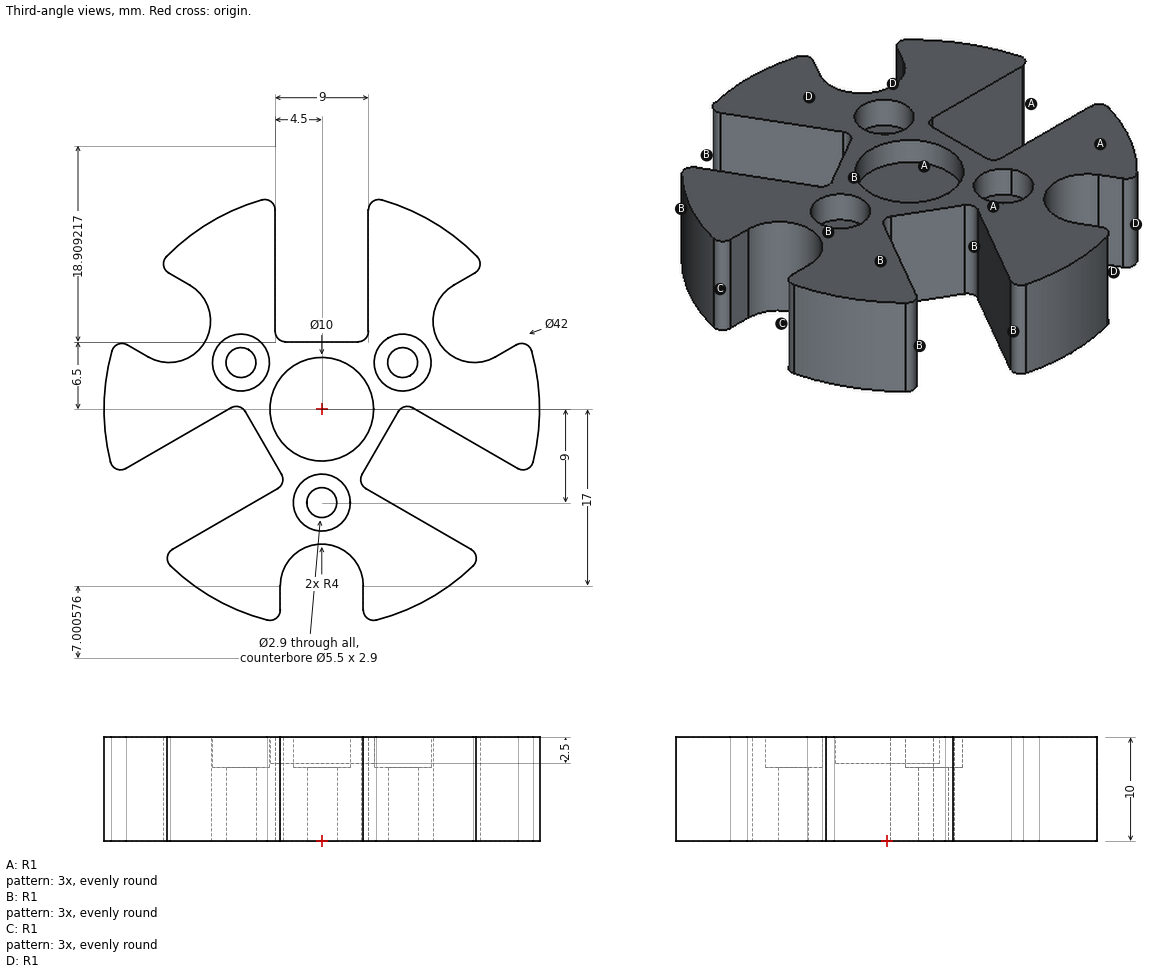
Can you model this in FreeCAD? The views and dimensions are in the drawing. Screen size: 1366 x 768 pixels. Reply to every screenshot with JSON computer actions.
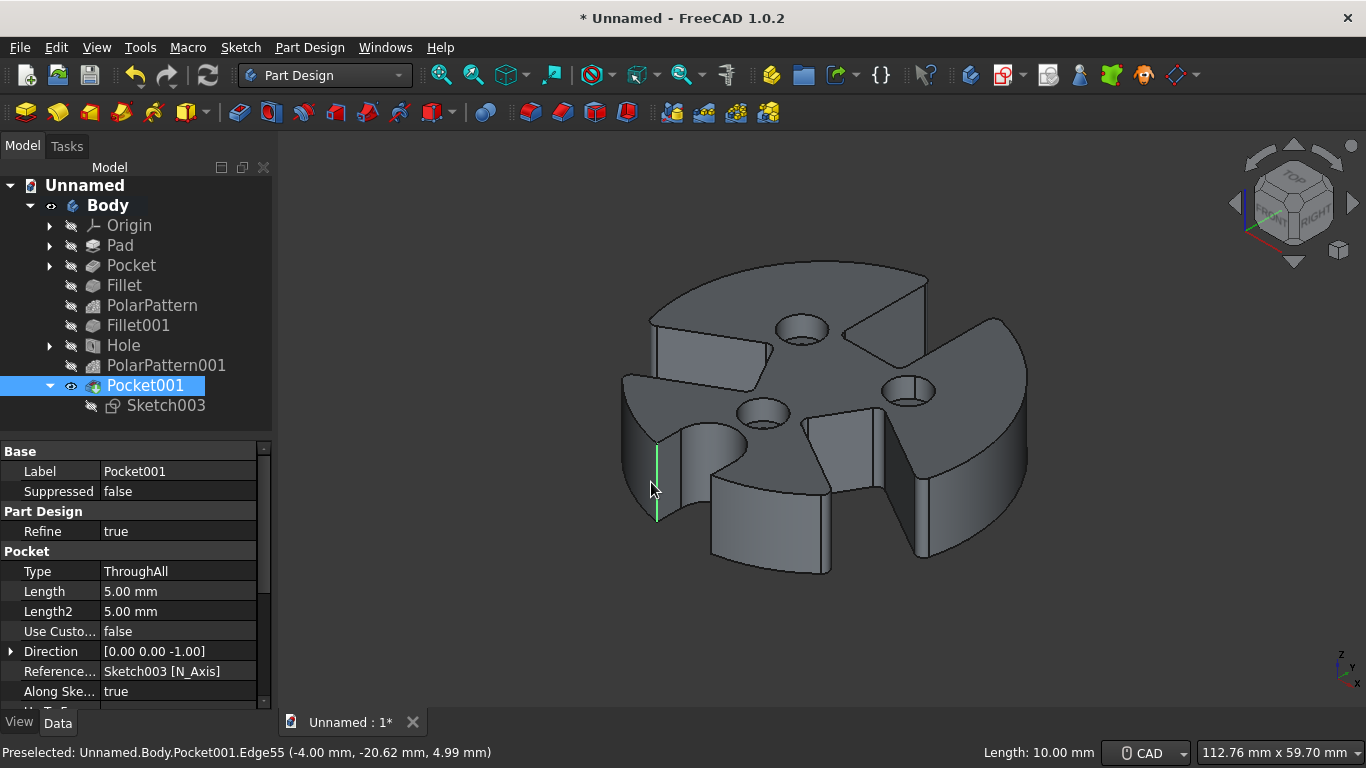
{"action": "key", "text": "2"}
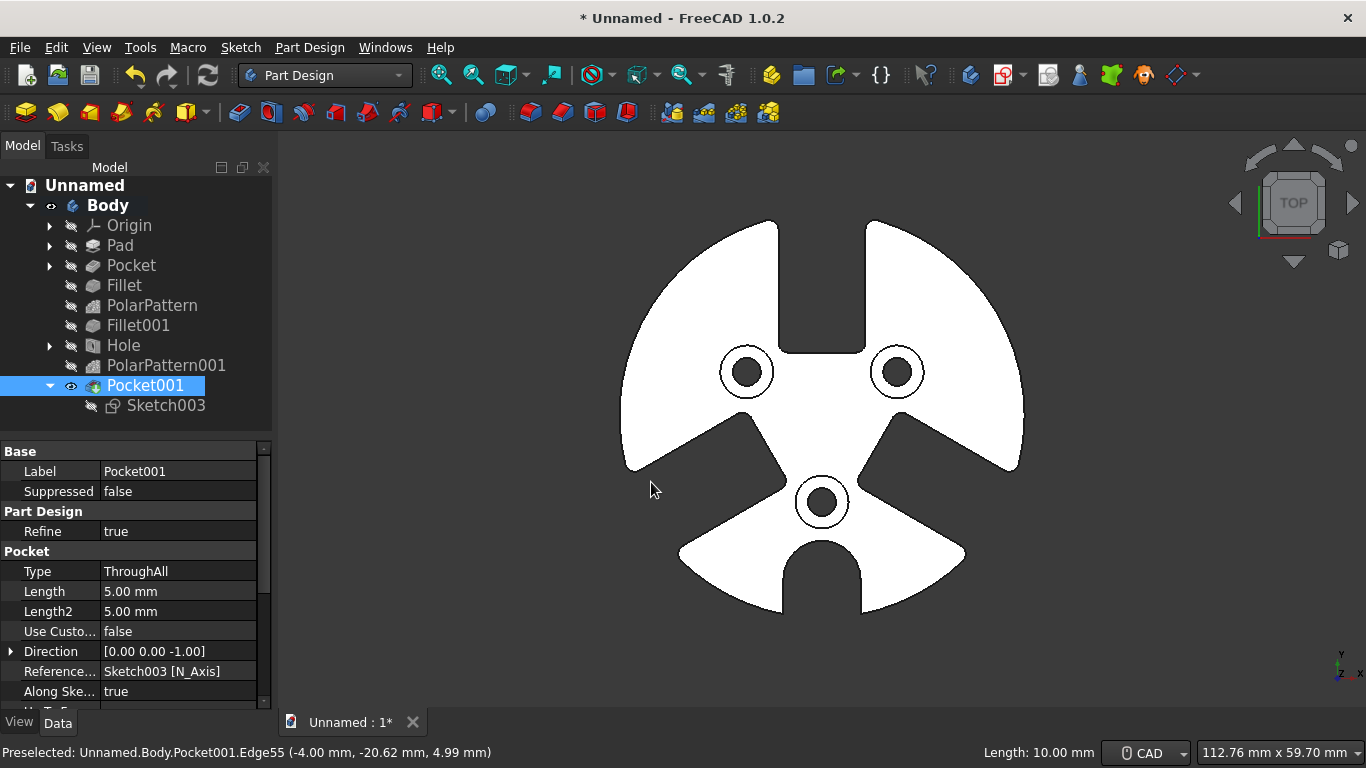
{"action": "key", "text": "0"}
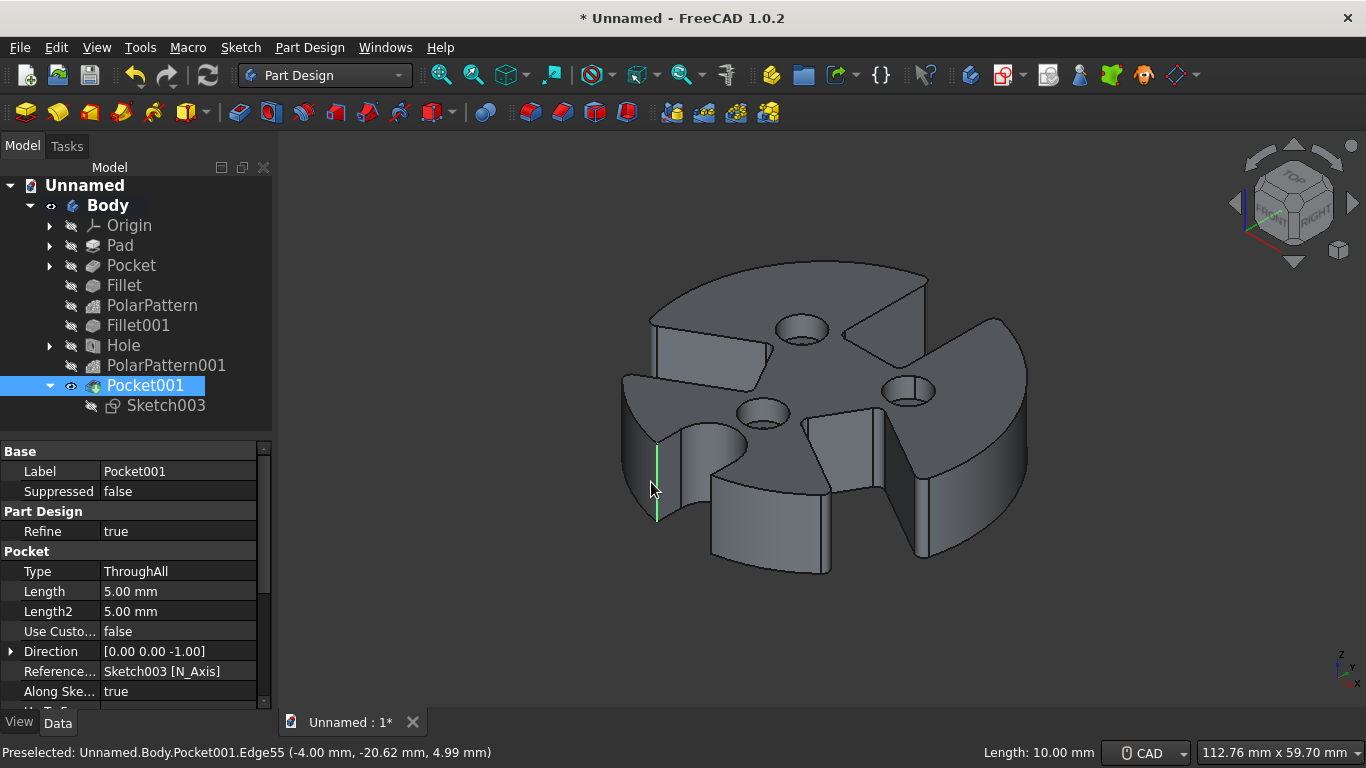
{"action": "key", "text": "1"}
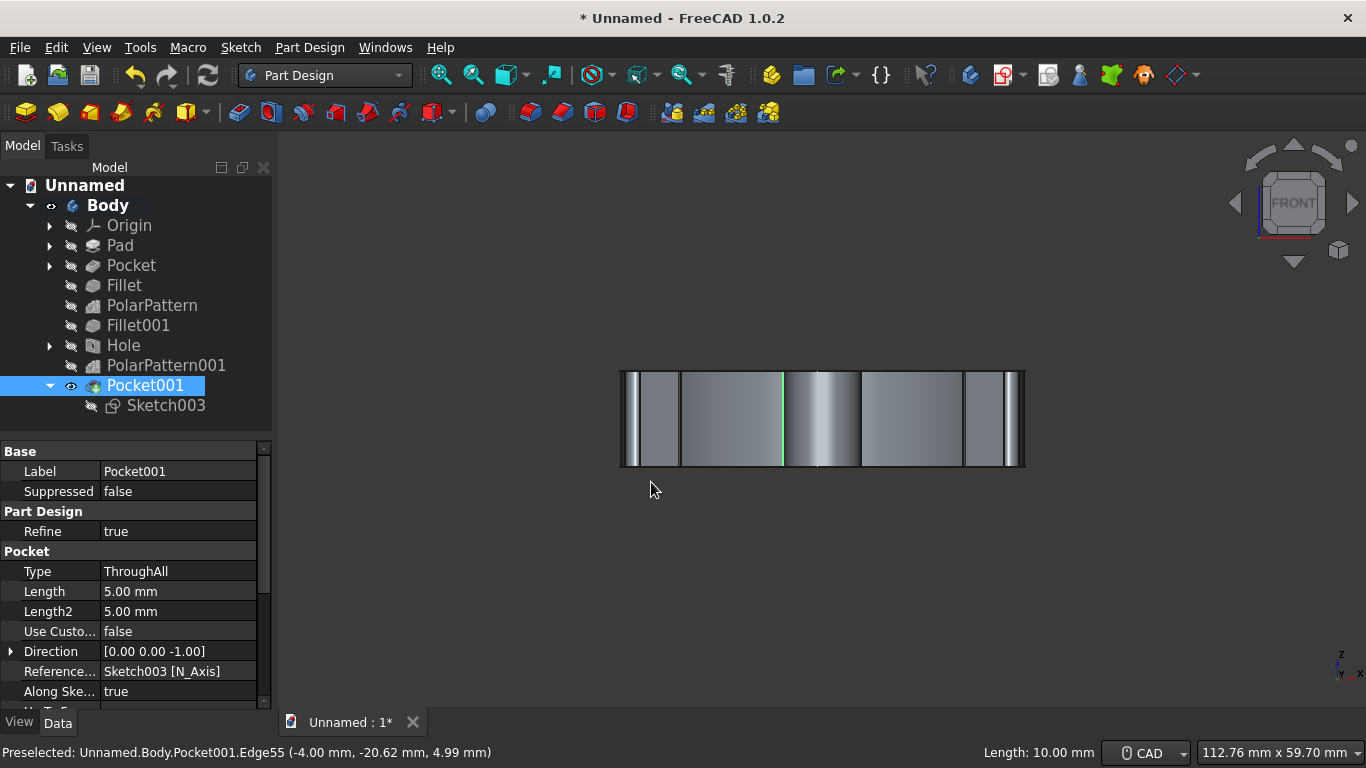
{"action": "left_click", "coordinate": [442, 76]}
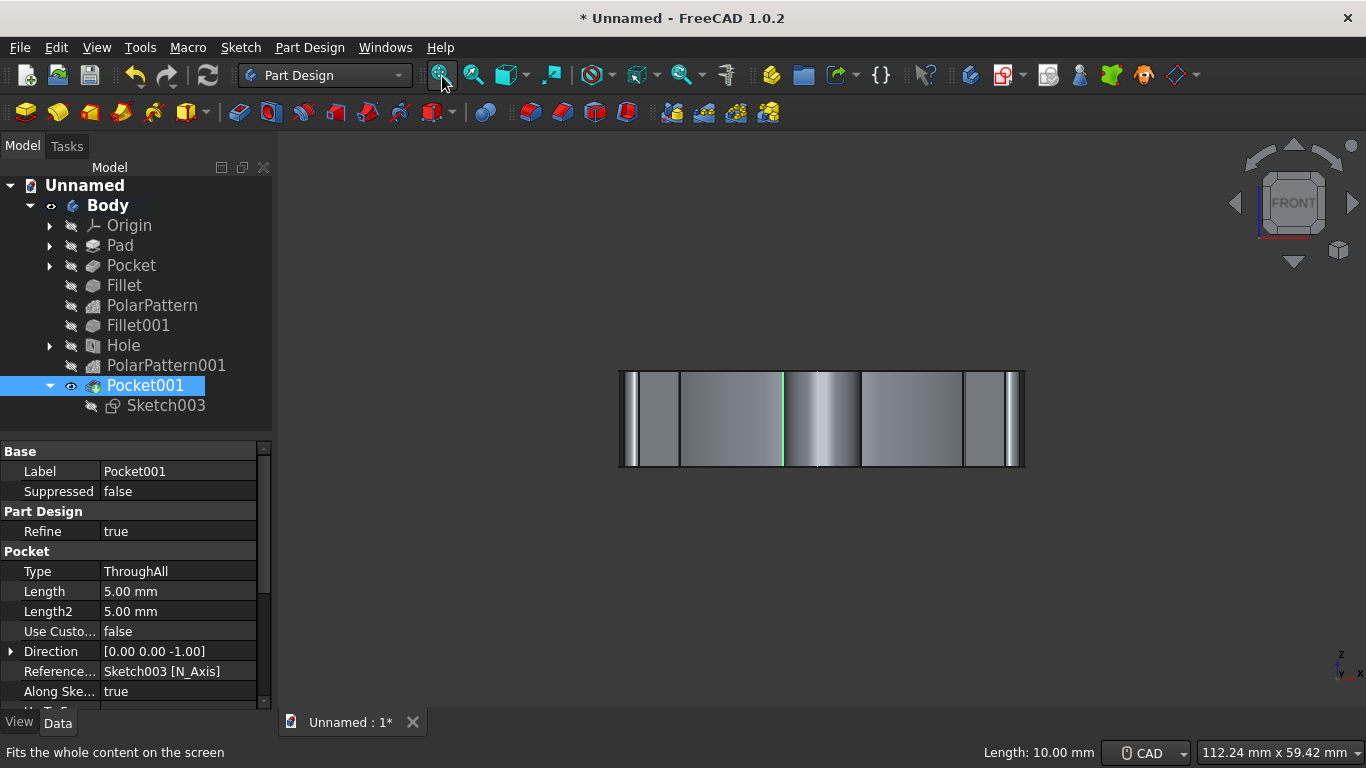
{"action": "left_click", "coordinate": [861, 418], "text": "ctrl"}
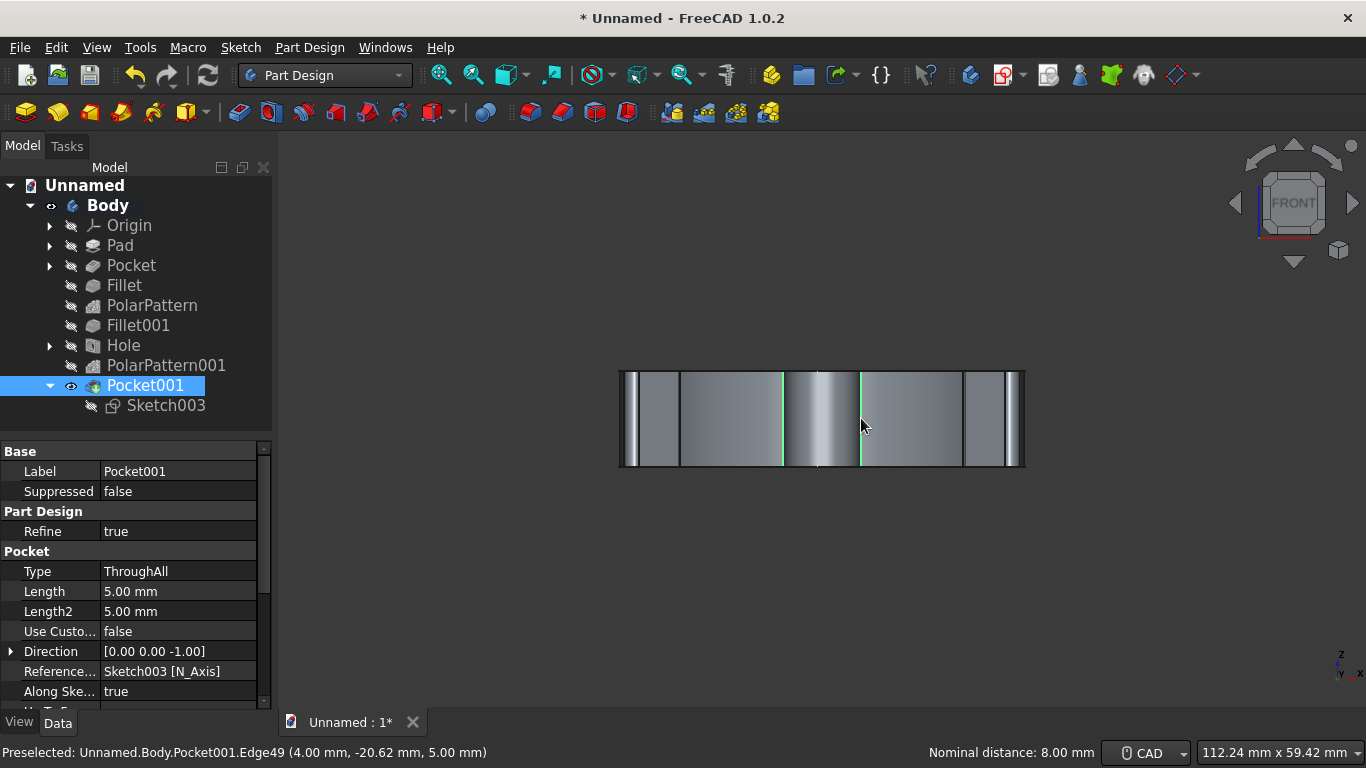
{"action": "left_click", "coordinate": [532, 112]}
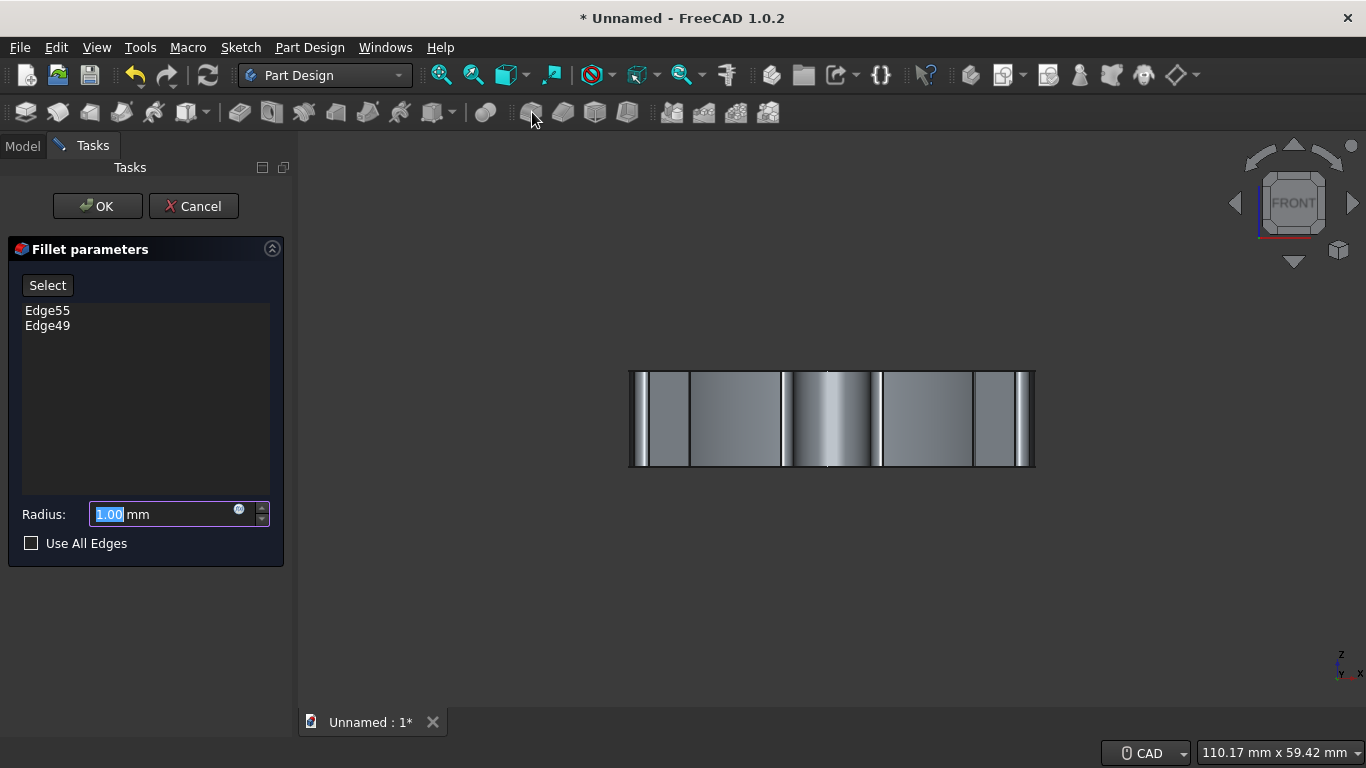
{"action": "type", "text": "1"}
{"action": "key", "text": "Tab"}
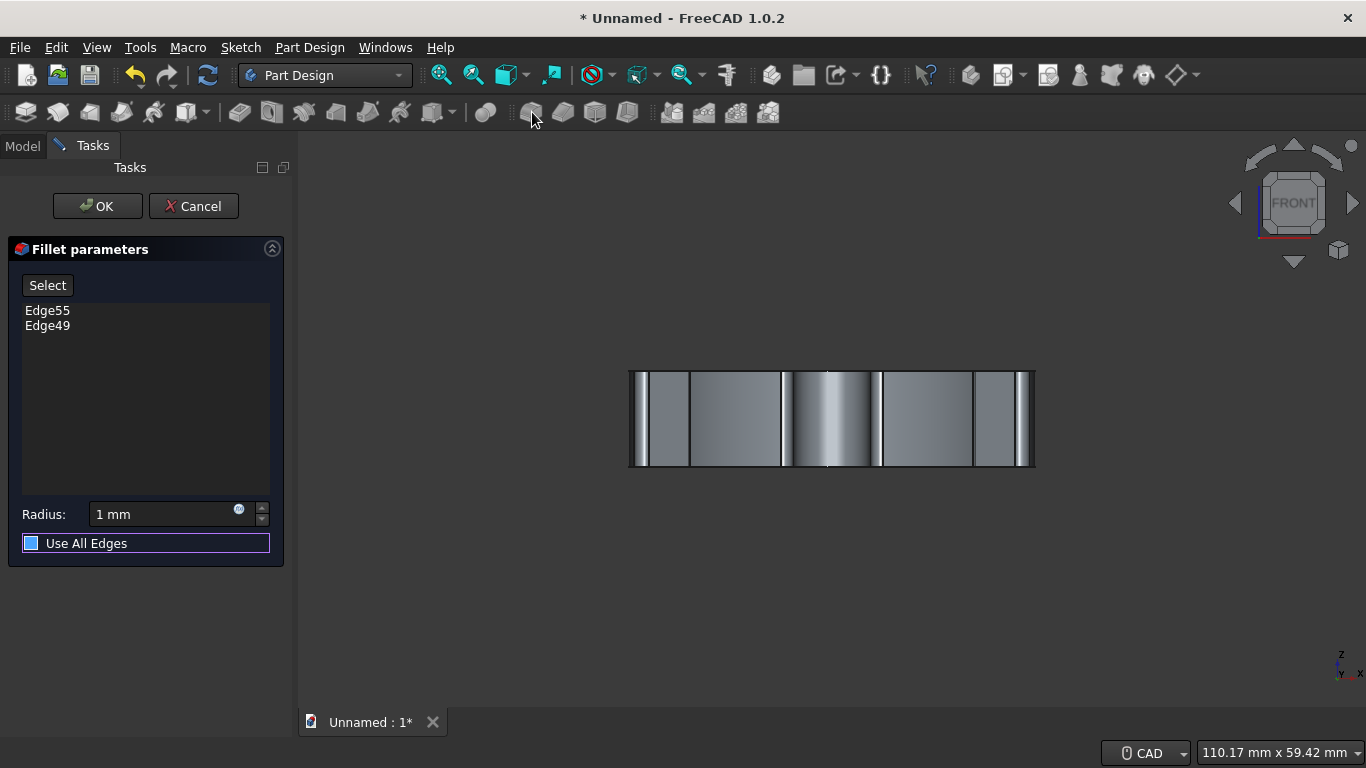
{"action": "left_click", "coordinate": [98, 206]}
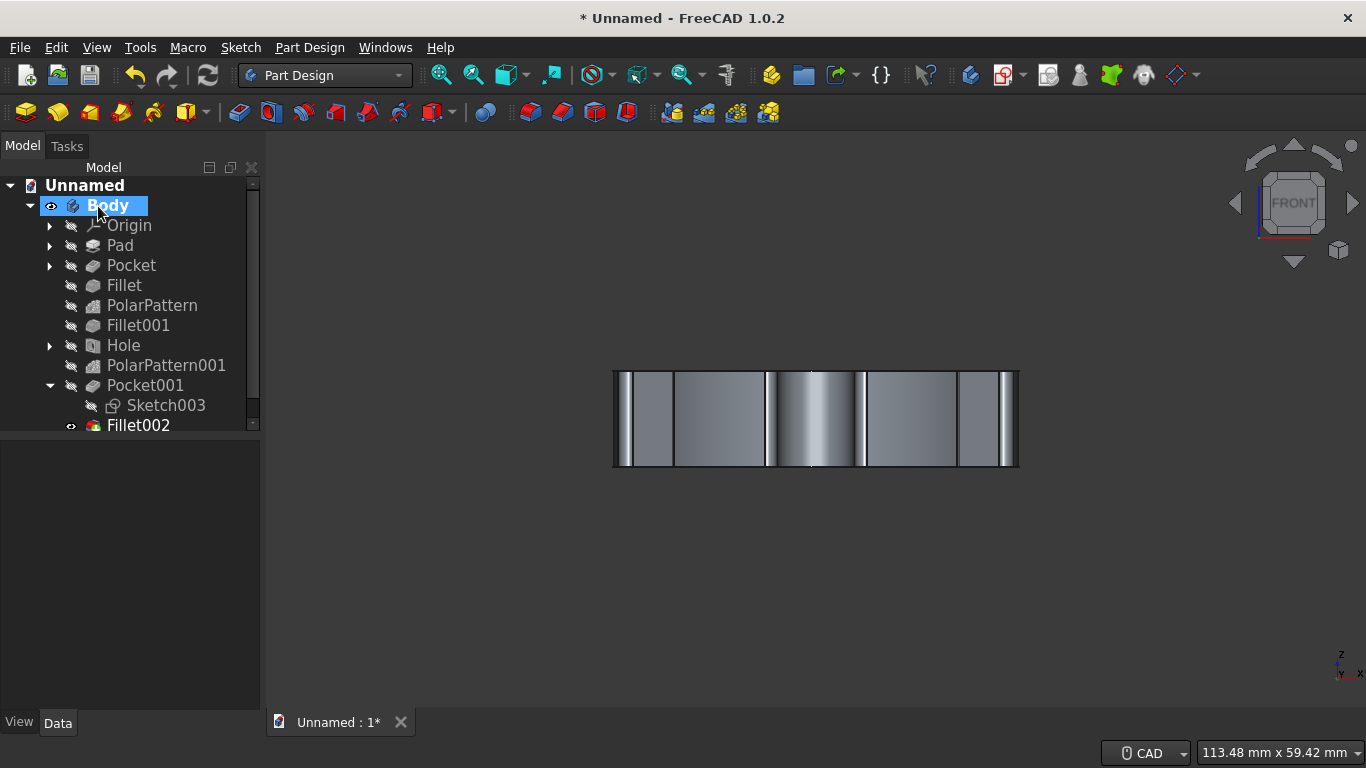
{"action": "left_click", "coordinate": [442, 76]}